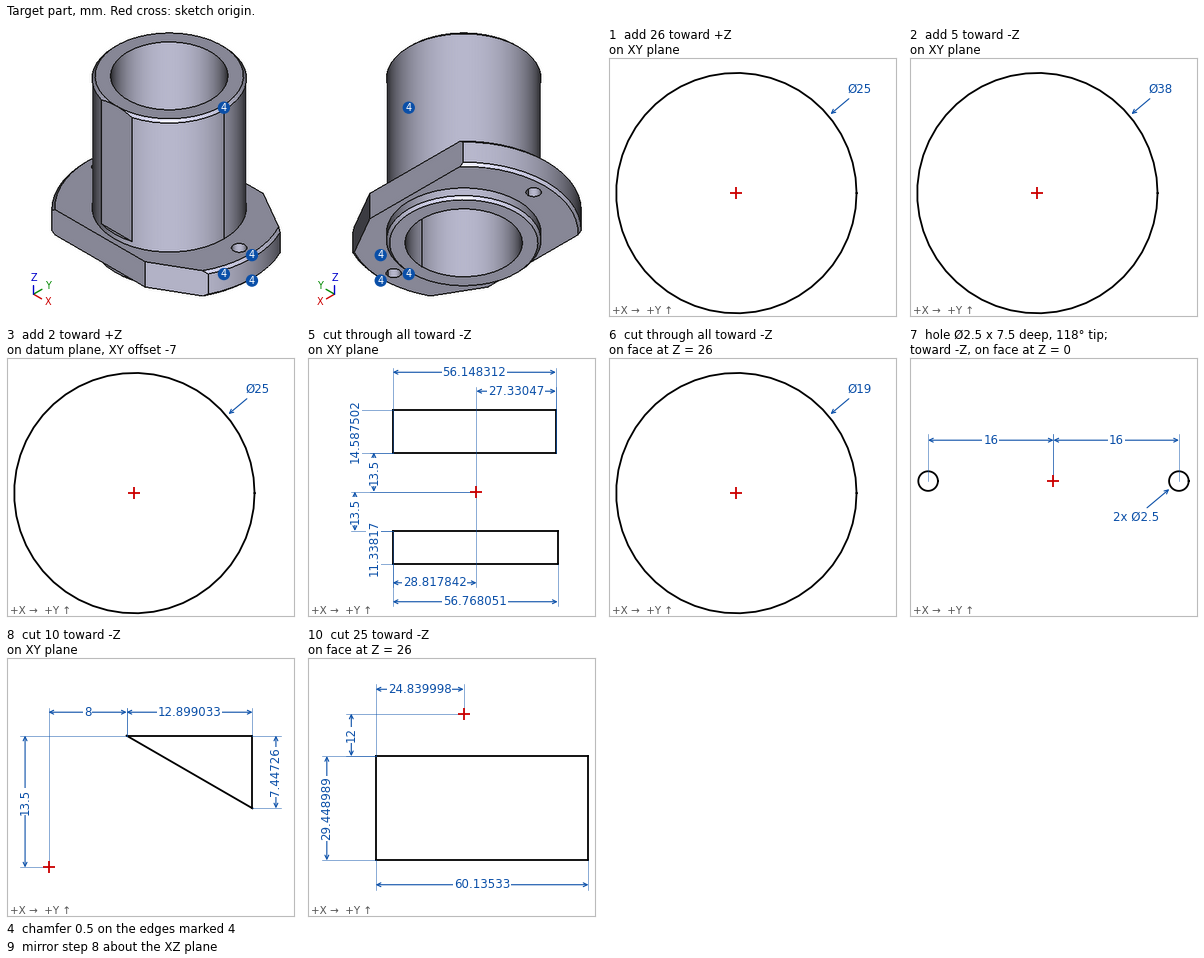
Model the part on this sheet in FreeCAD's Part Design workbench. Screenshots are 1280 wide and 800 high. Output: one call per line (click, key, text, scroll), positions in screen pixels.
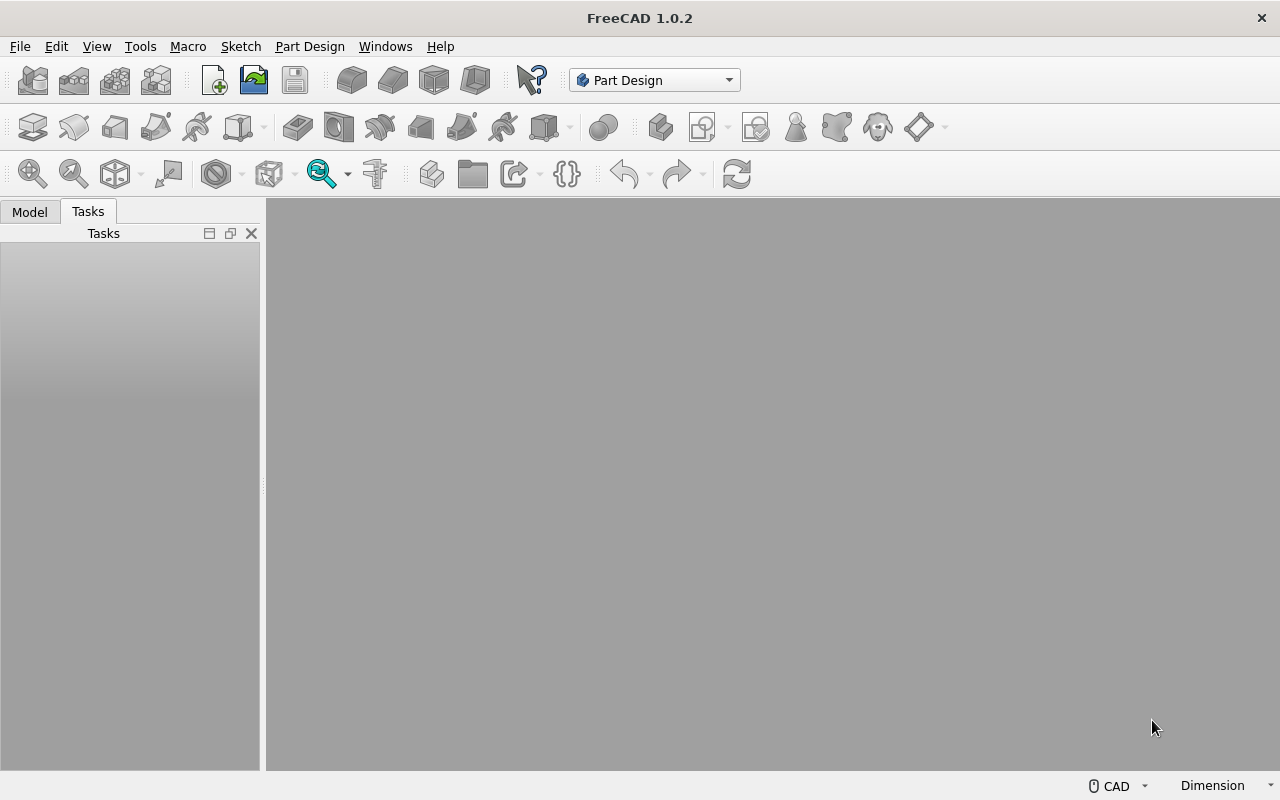
click(213, 80)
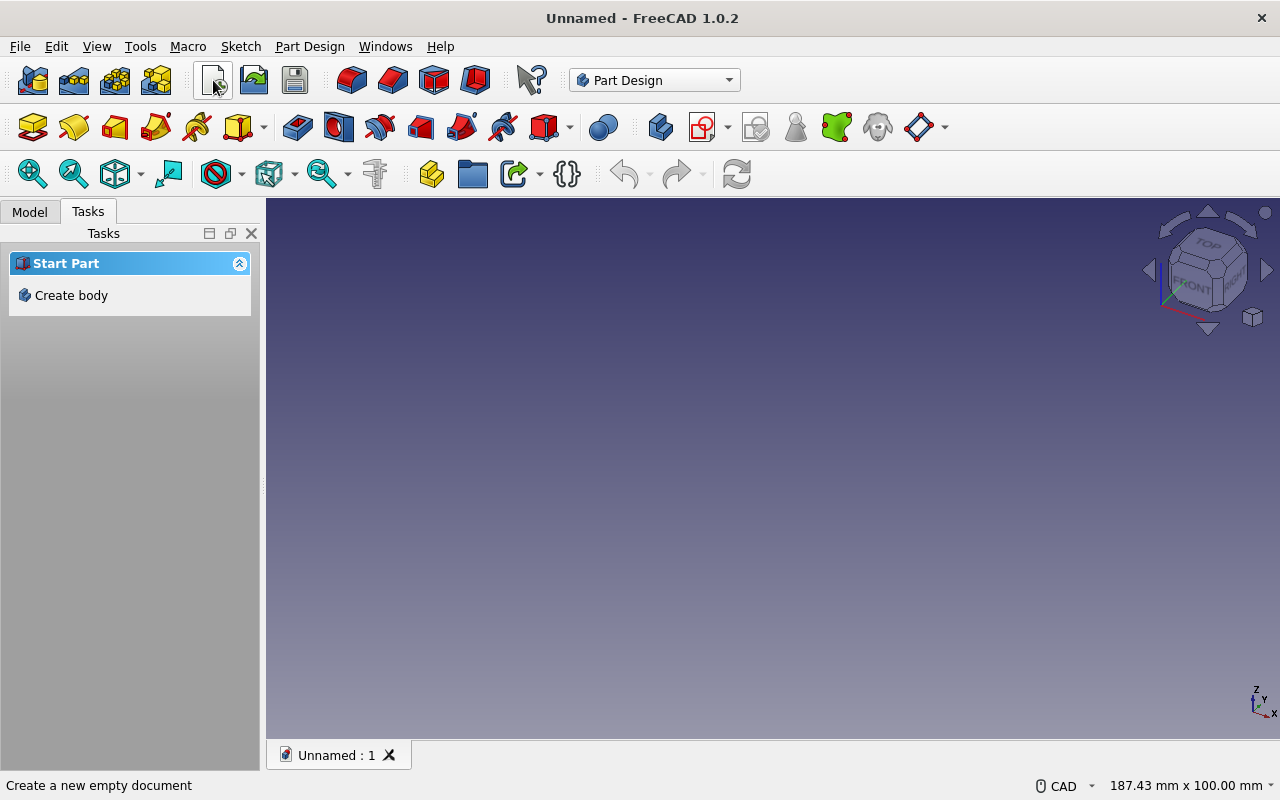
click(702, 128)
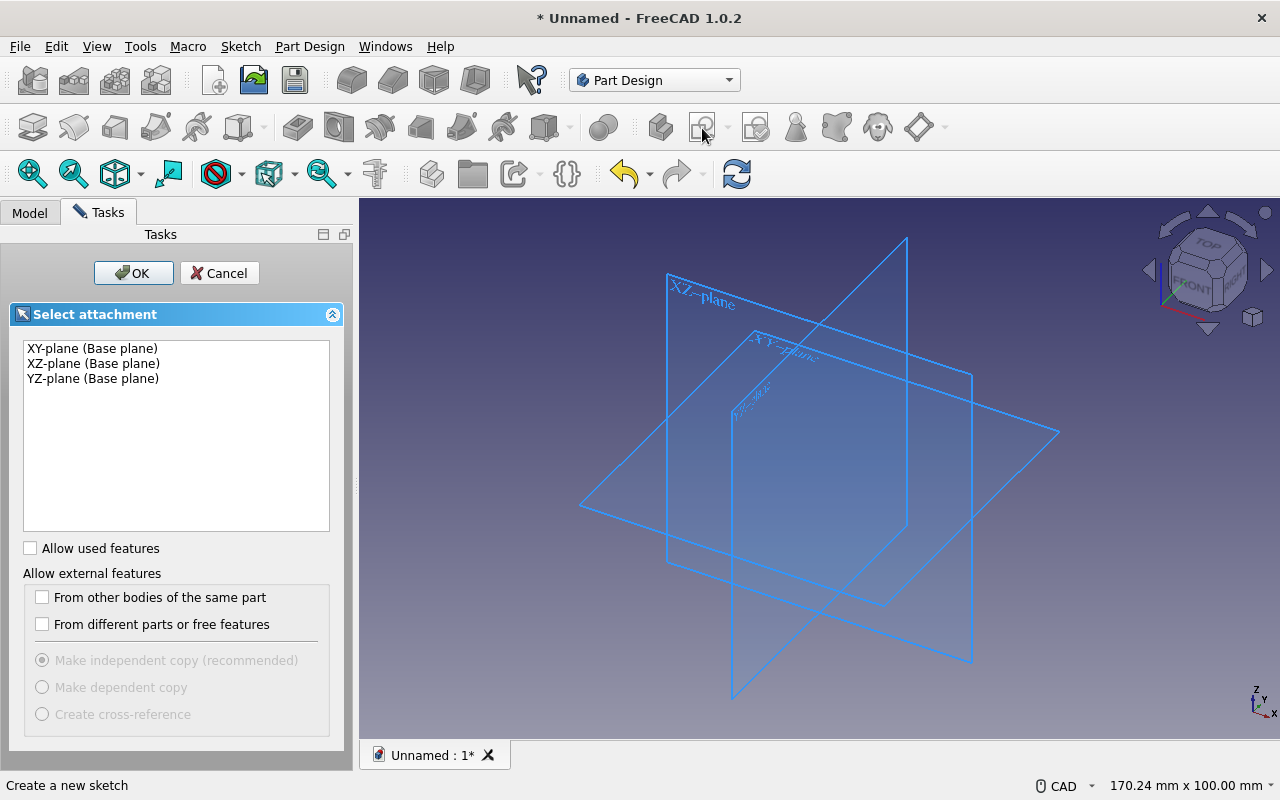
click(84, 348)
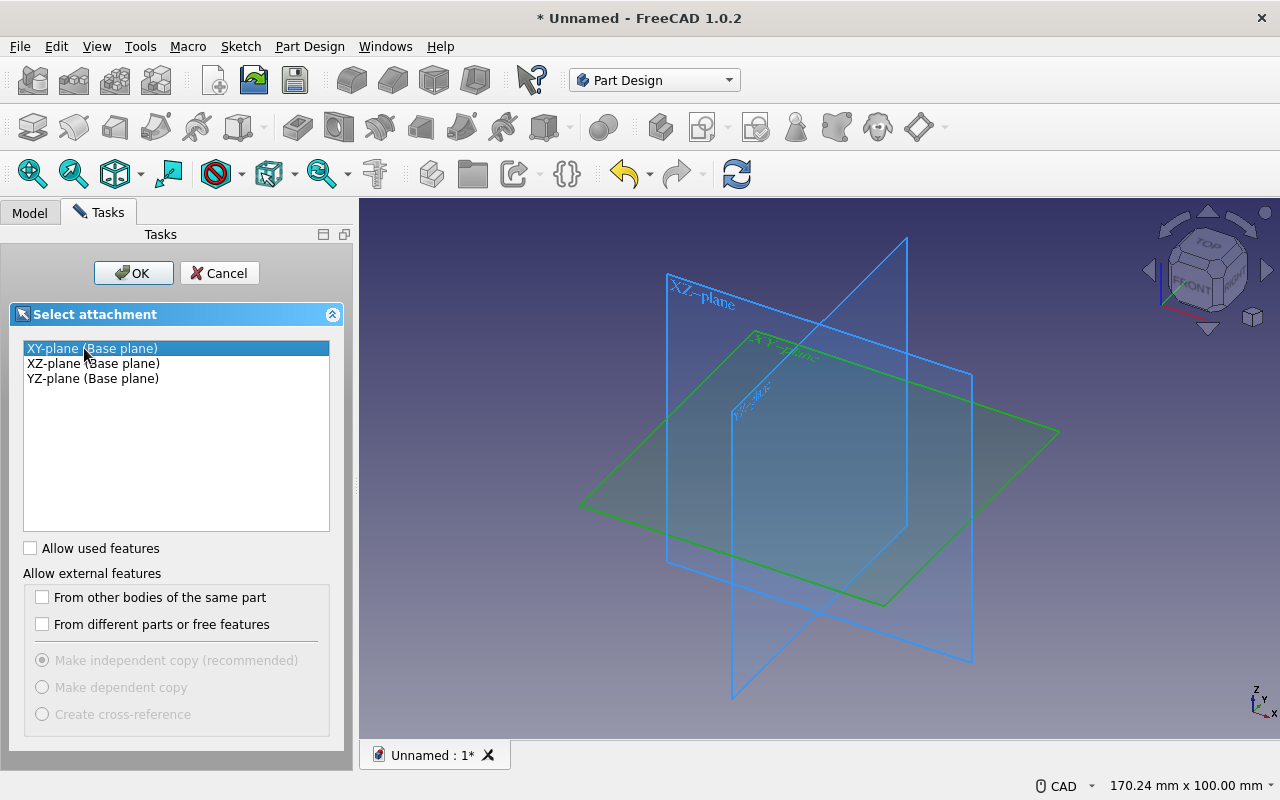
click(134, 273)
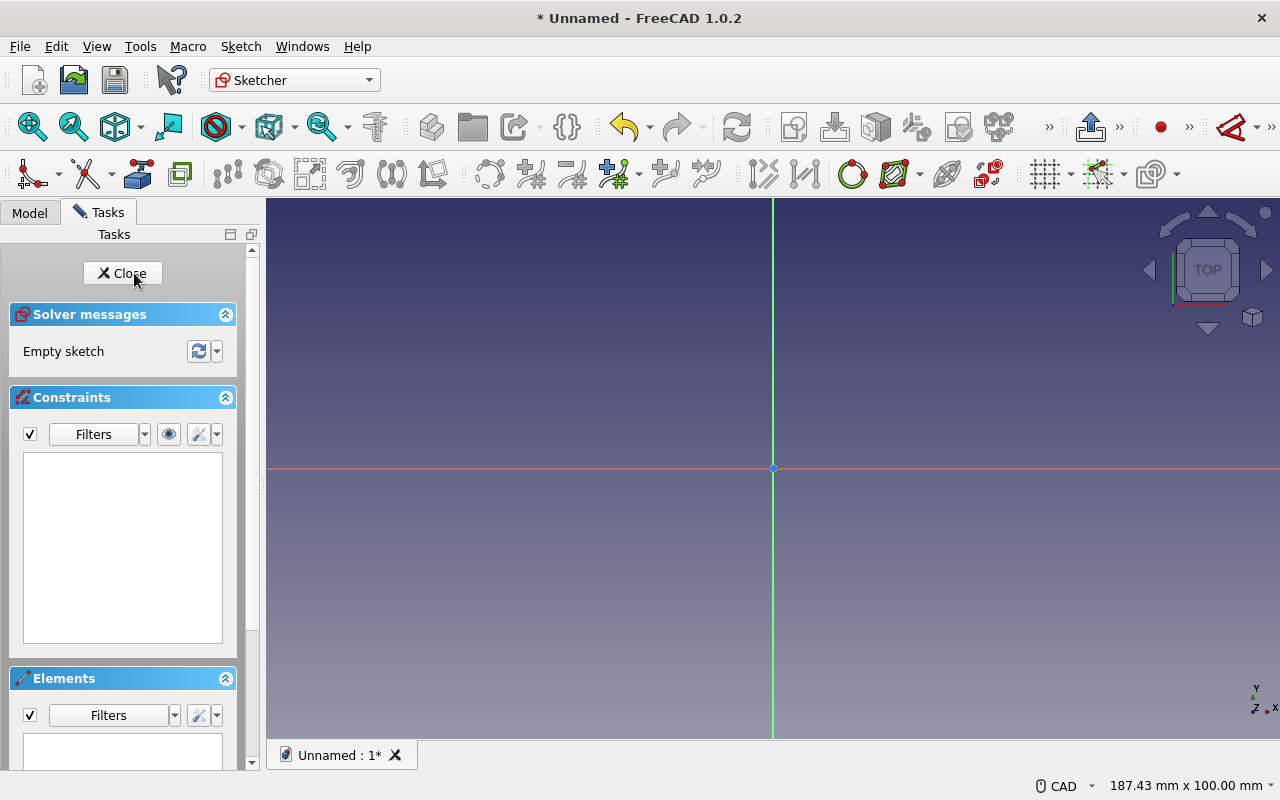
scroll(813, 468, up, 5)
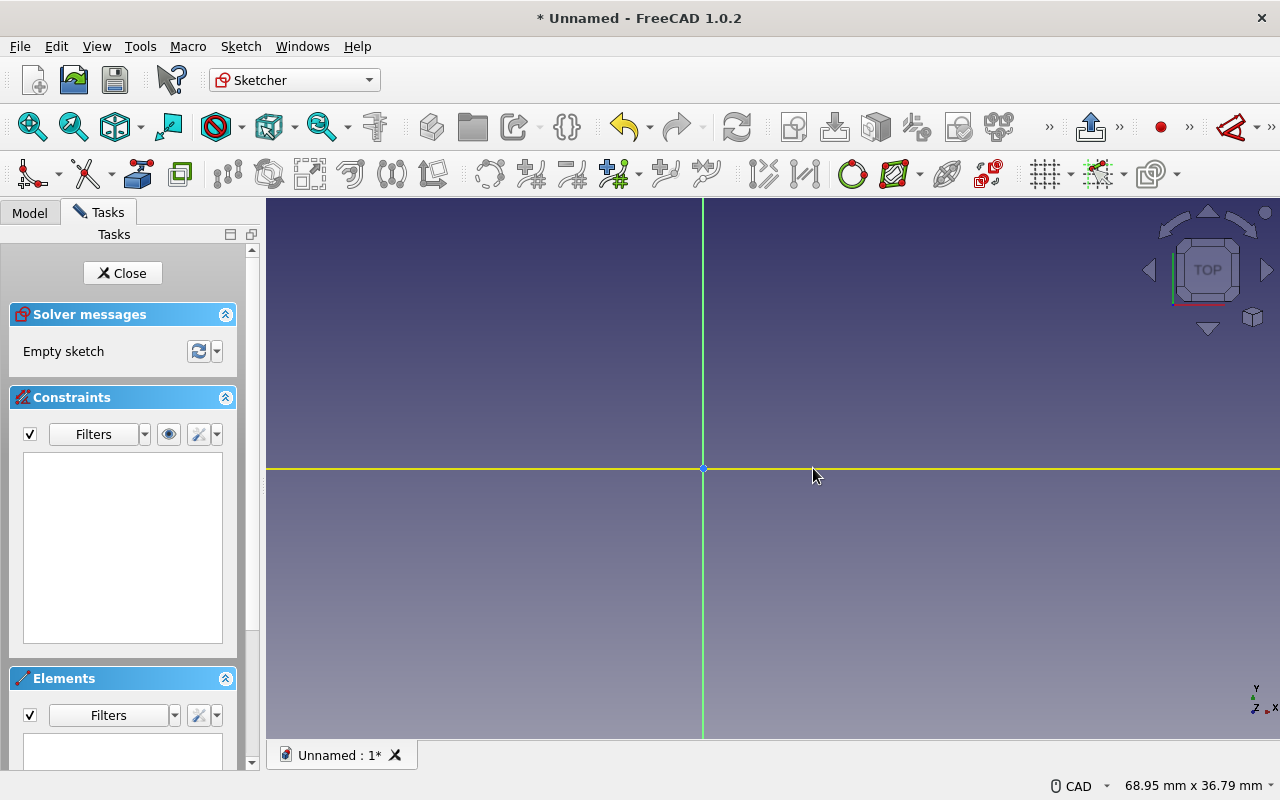
key(g)
key(c)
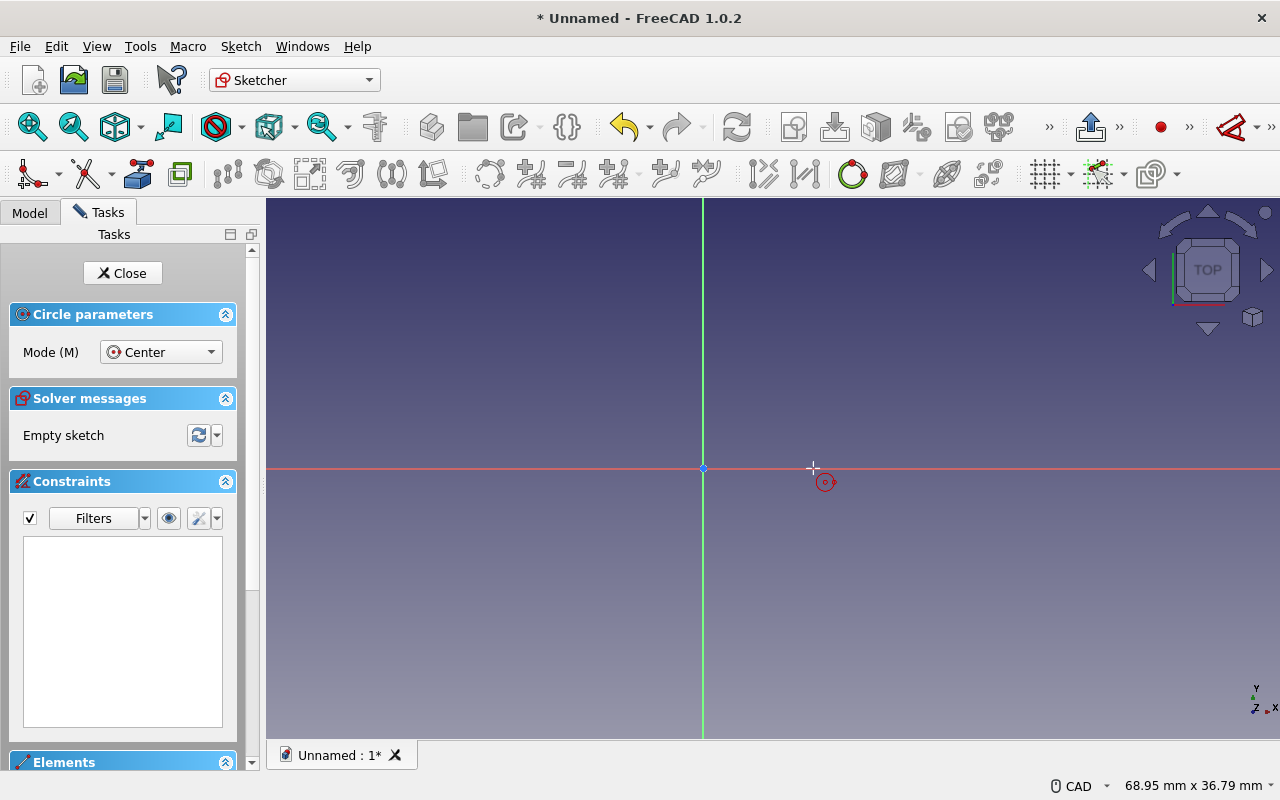
click(703, 468)
click(833, 339)
key(Escape)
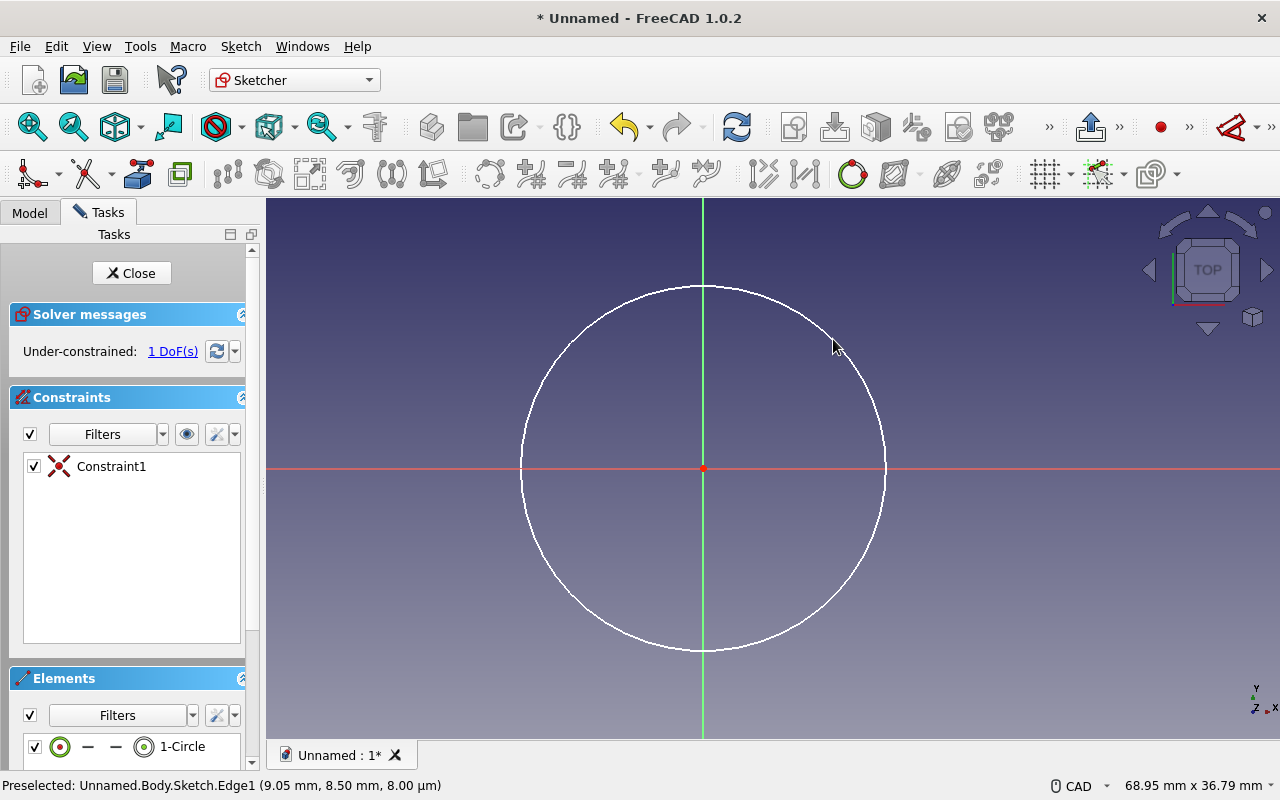
click(832, 339)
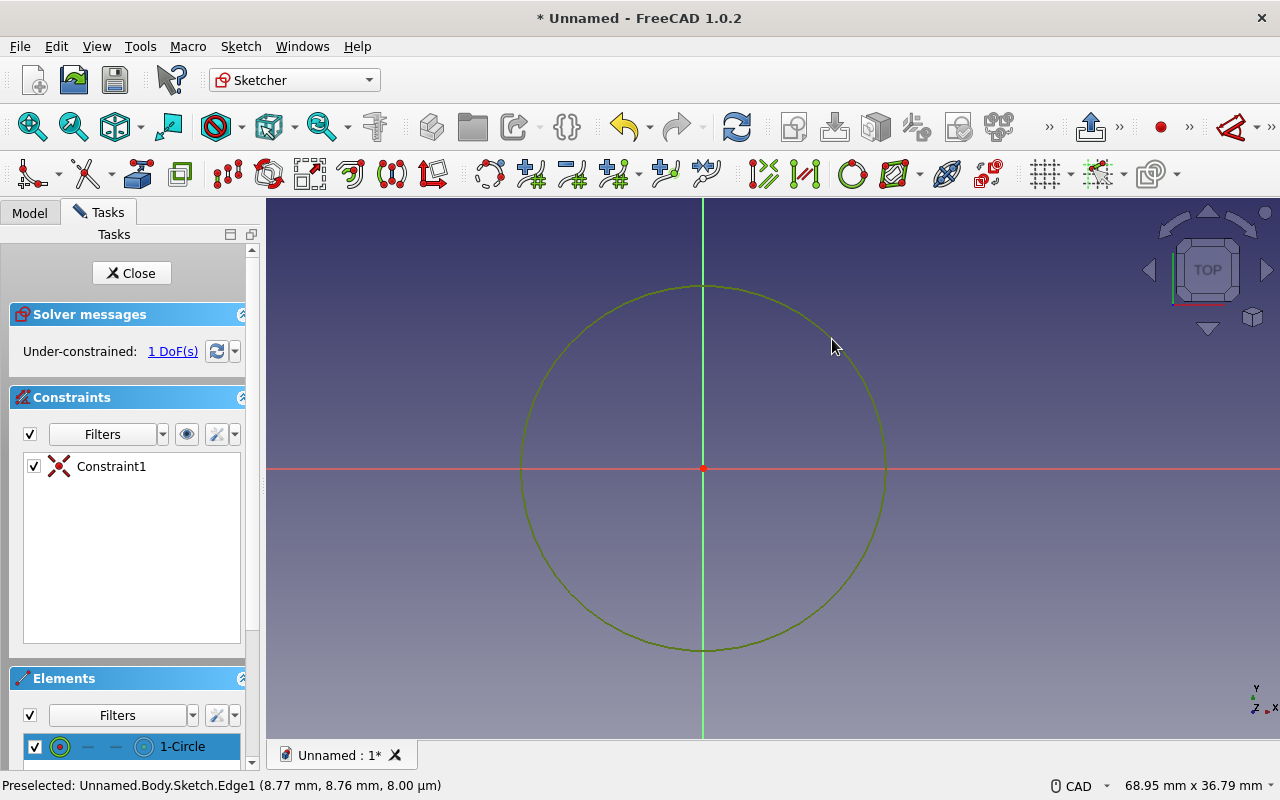
click(1256, 128)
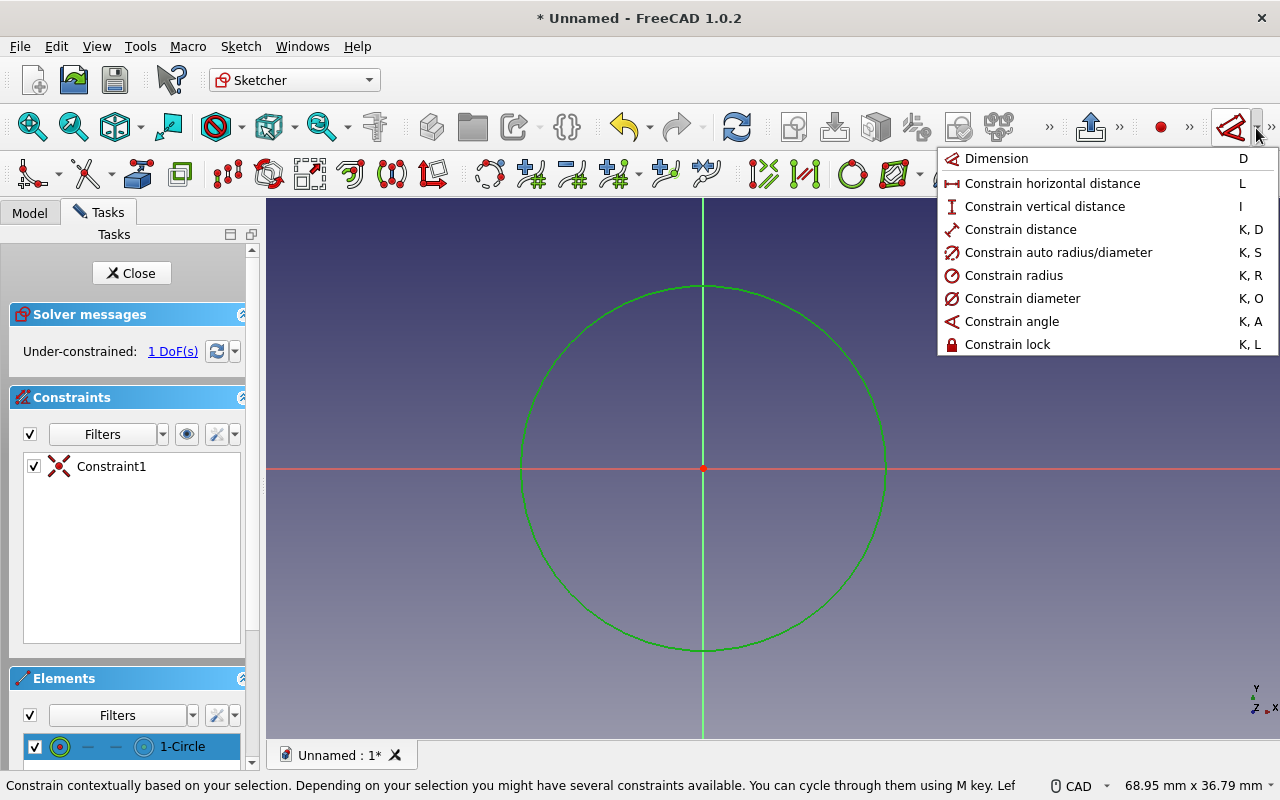
click(1108, 298)